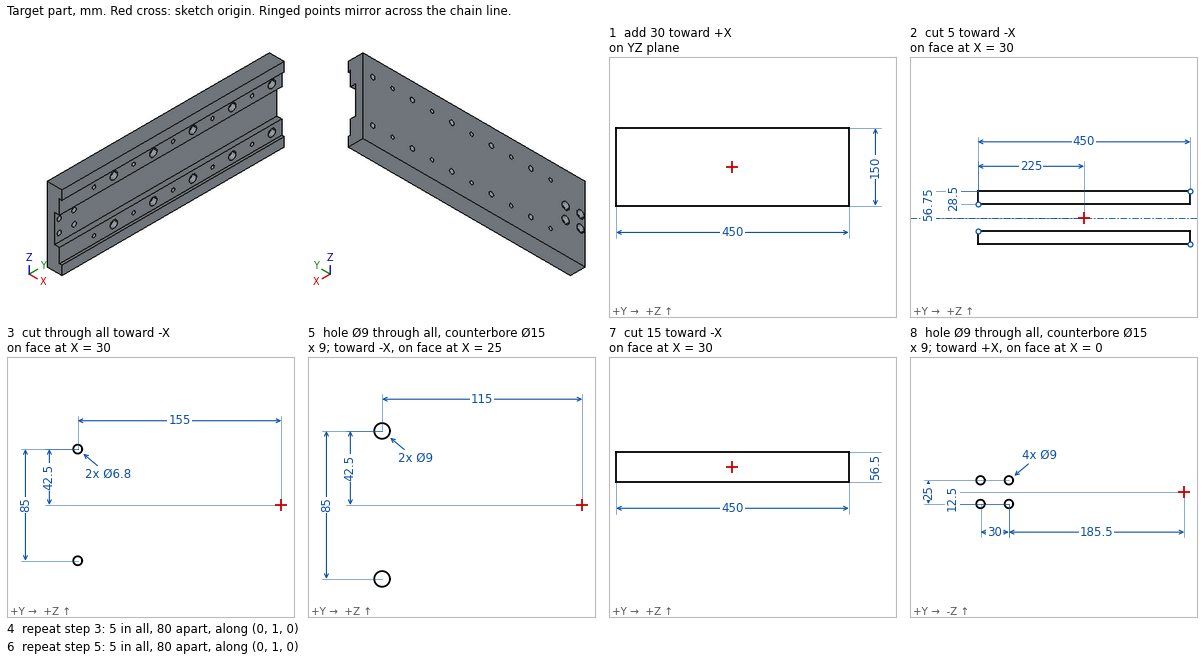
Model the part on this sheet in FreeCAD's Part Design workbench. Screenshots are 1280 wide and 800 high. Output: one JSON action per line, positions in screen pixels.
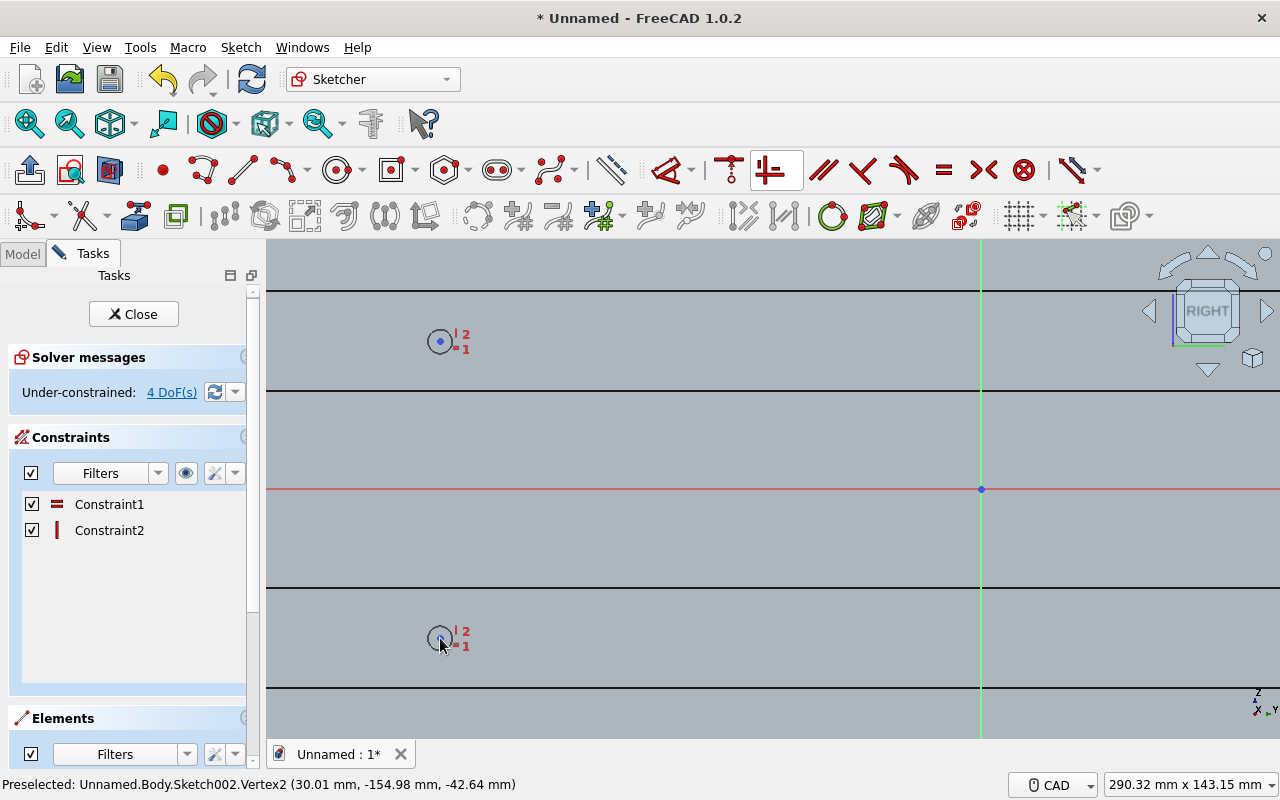
{"action": "left_click", "coordinate": [666, 170]}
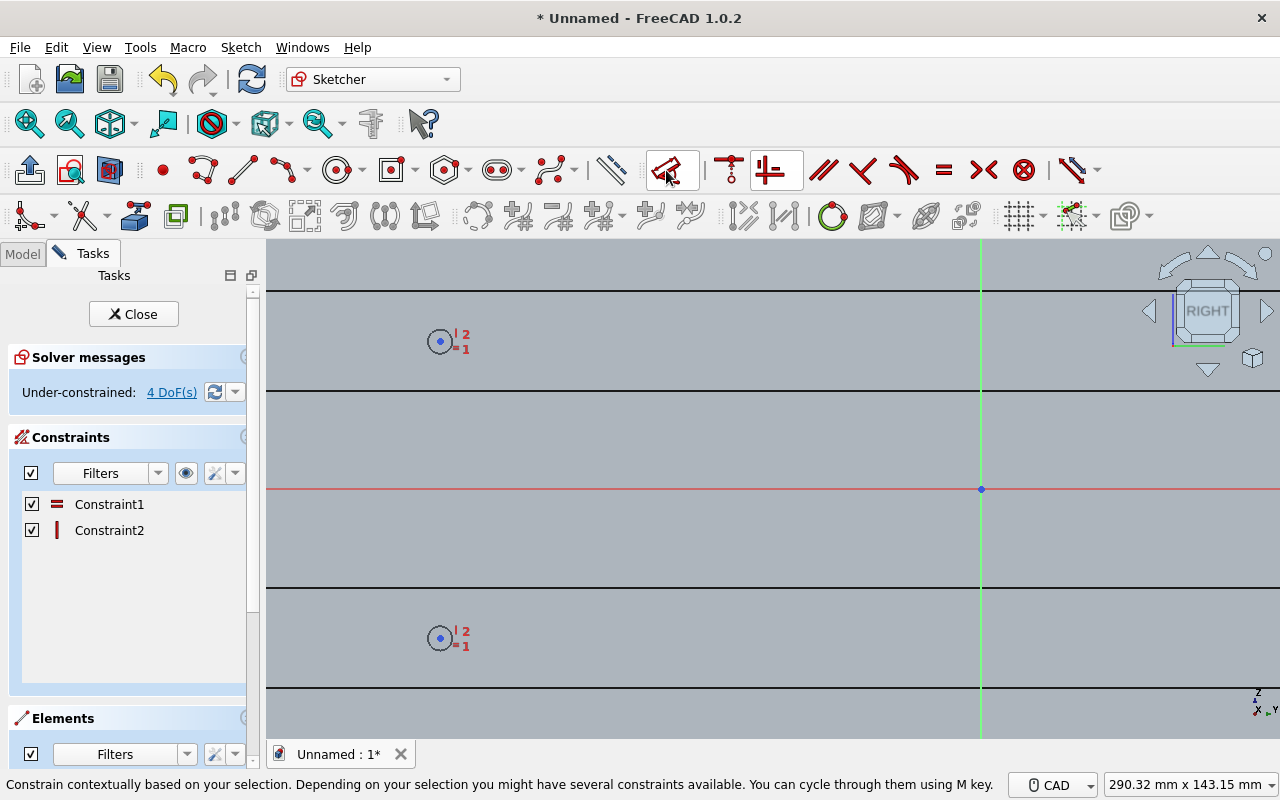
{"action": "scroll", "coordinate": [449, 333], "scroll_direction": "up", "scroll_amount": 3}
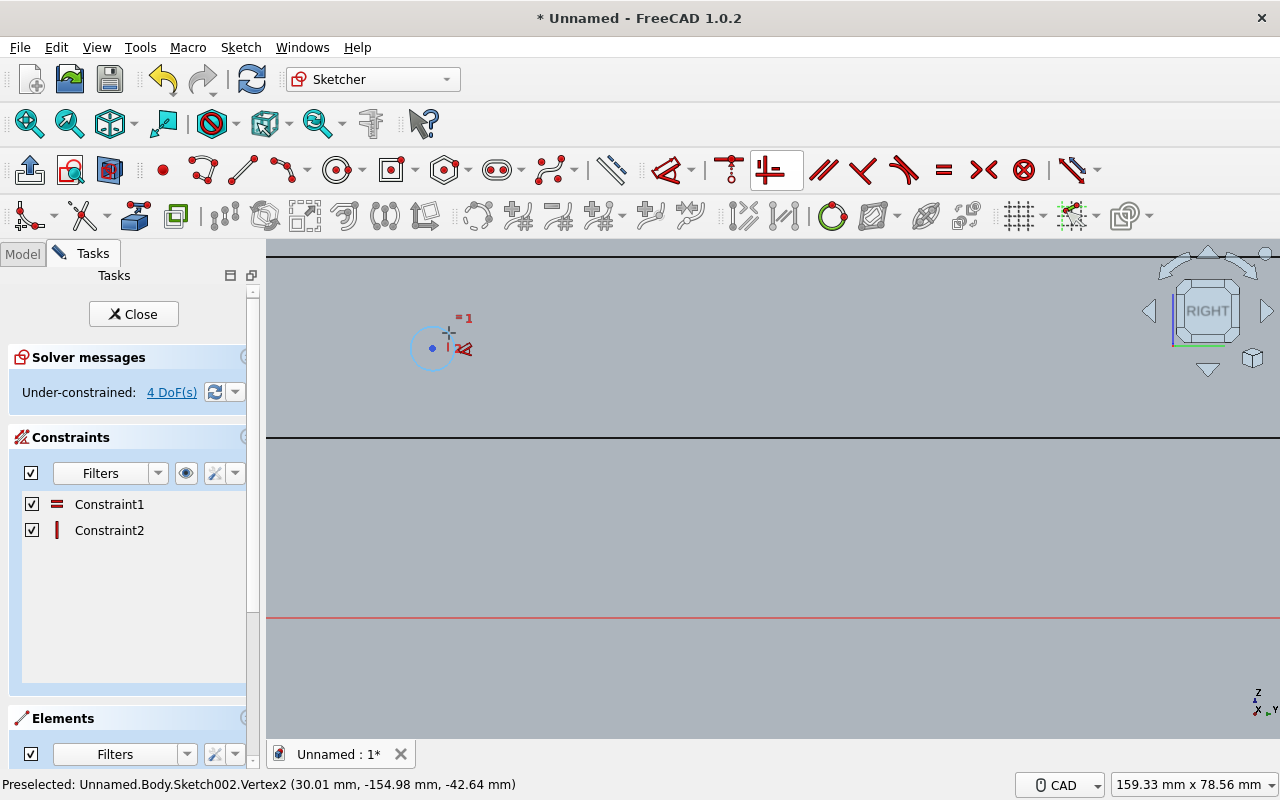
{"action": "left_click", "coordinate": [448, 333]}
{"action": "left_click", "coordinate": [470, 310]}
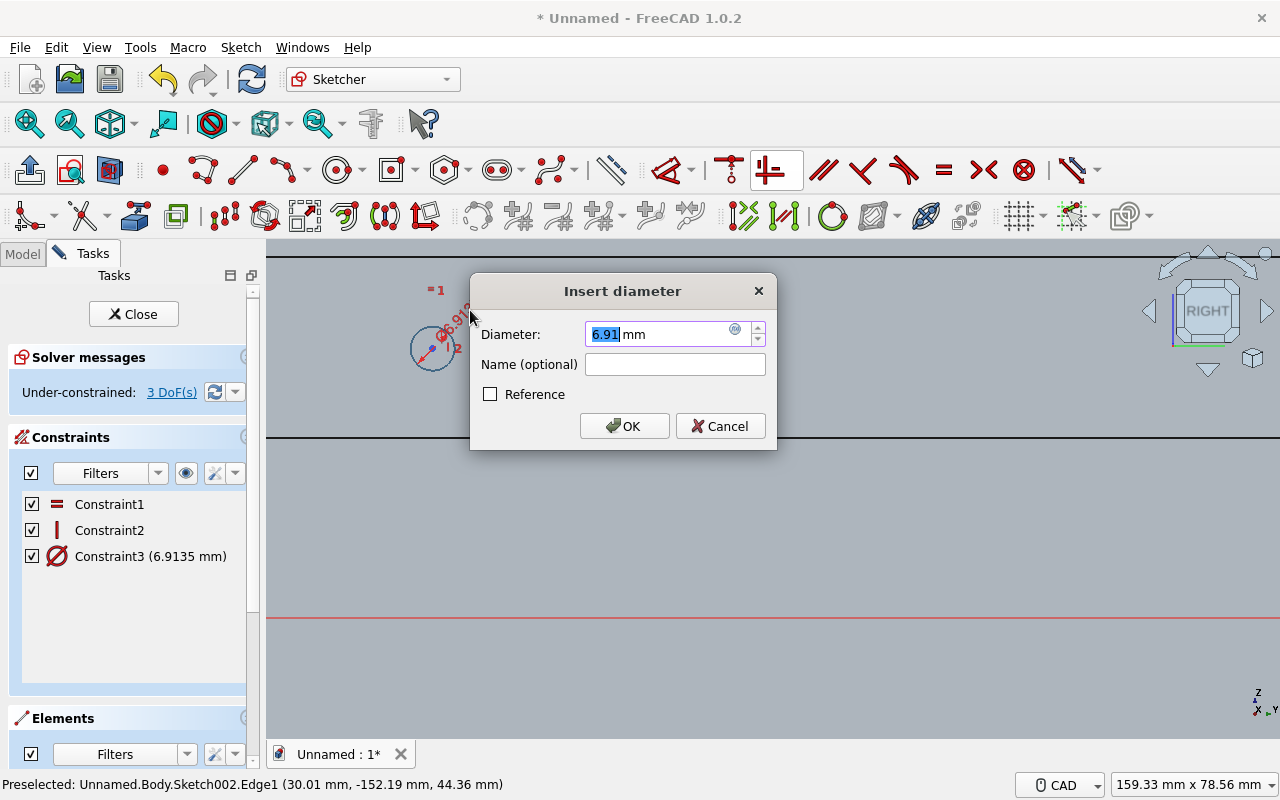
{"action": "type", "text": "6.8"}
{"action": "key", "text": "Return"}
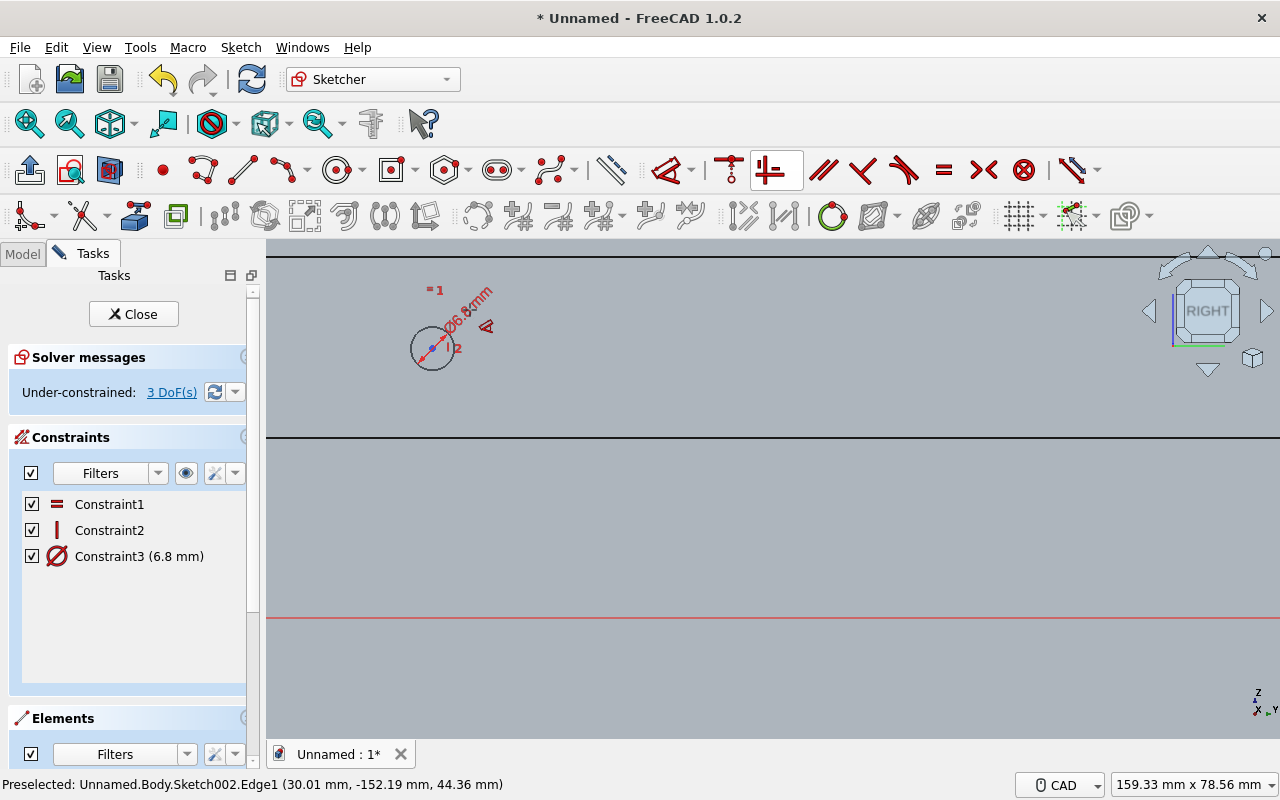
{"action": "left_click", "coordinate": [433, 349]}
{"action": "left_click", "coordinate": [774, 315]}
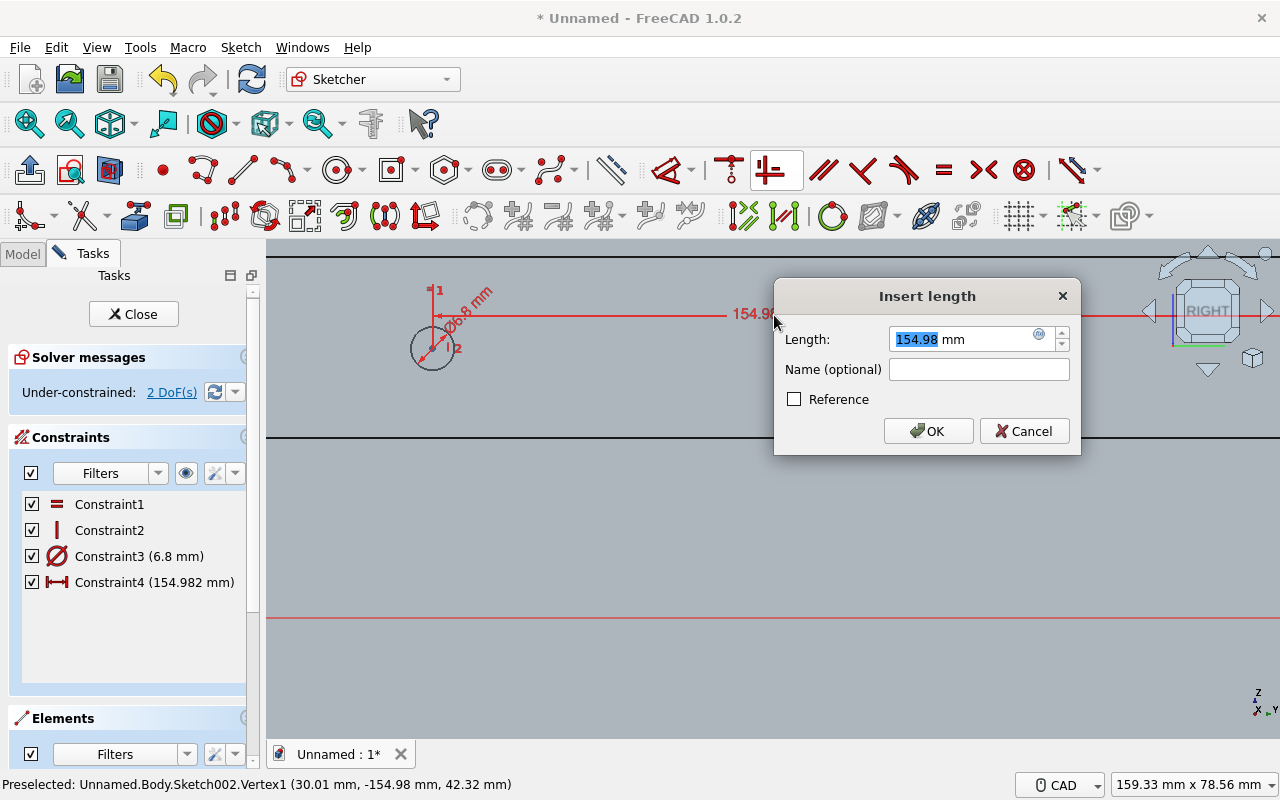
{"action": "type", "text": "155"}
{"action": "key", "text": "Return"}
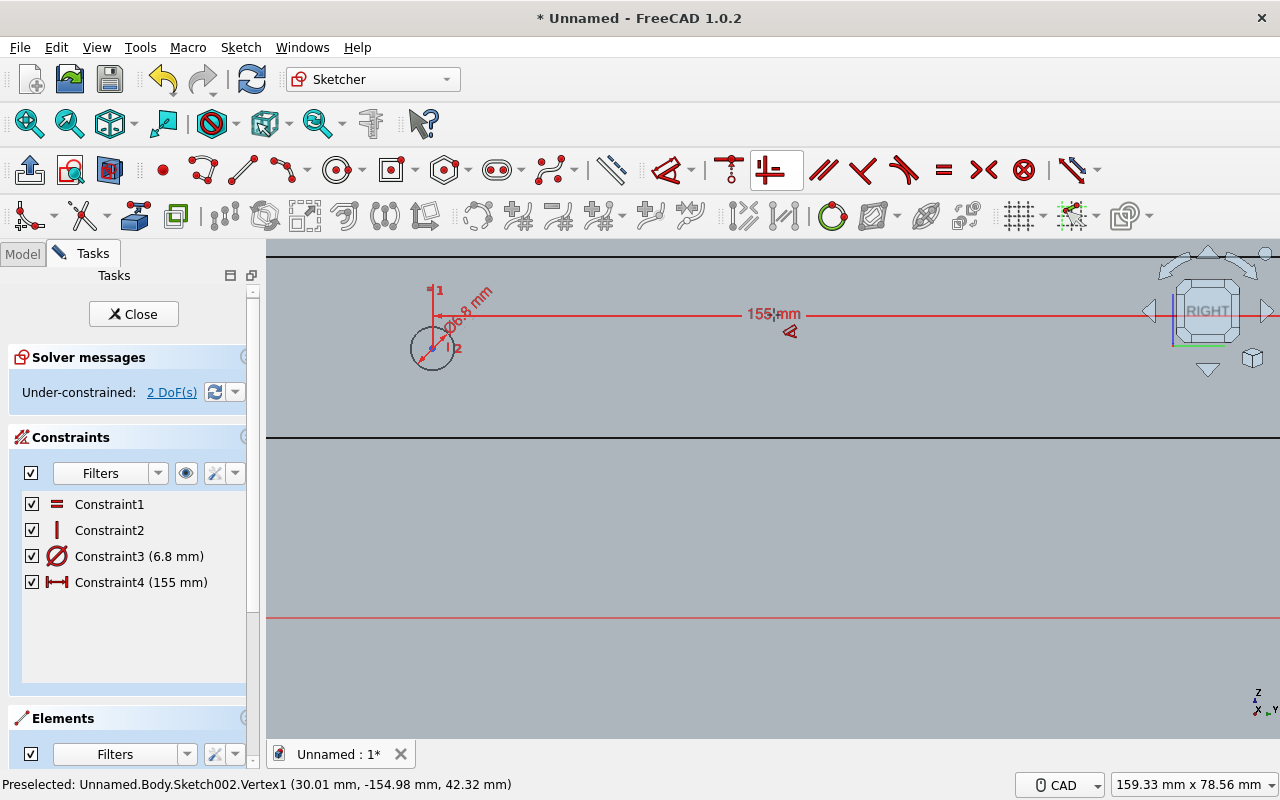
{"action": "left_click", "coordinate": [433, 349]}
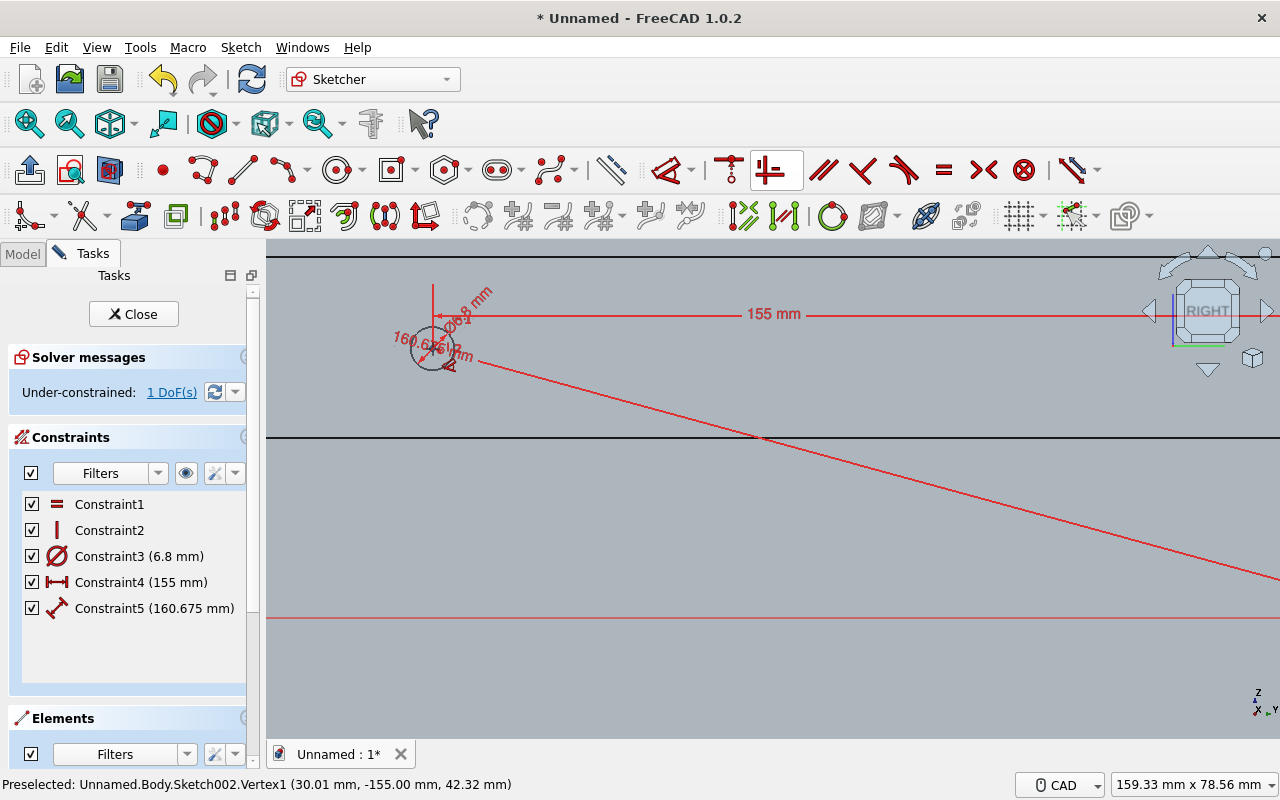
{"action": "scroll", "coordinate": [449, 332], "scroll_direction": "down", "scroll_amount": 3}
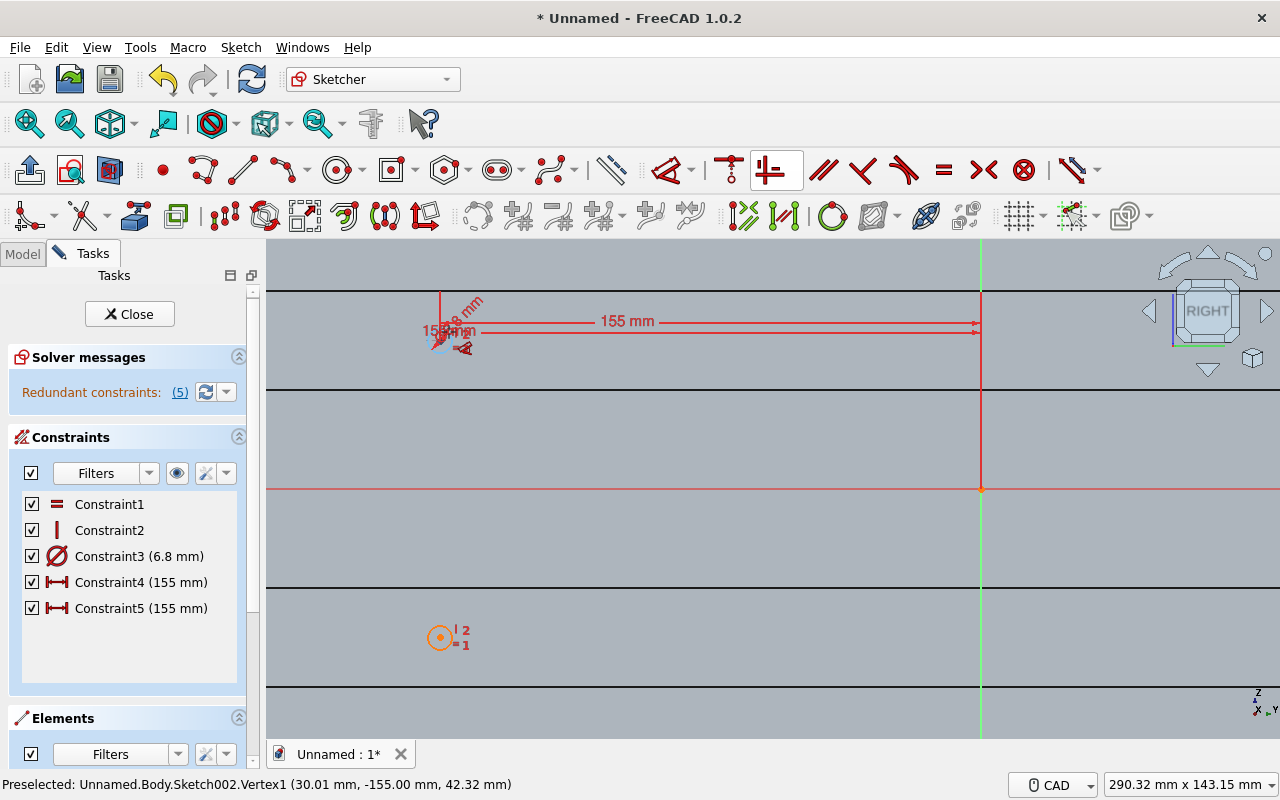
{"action": "left_click", "coordinate": [440, 638]}
{"action": "left_click", "coordinate": [406, 421]}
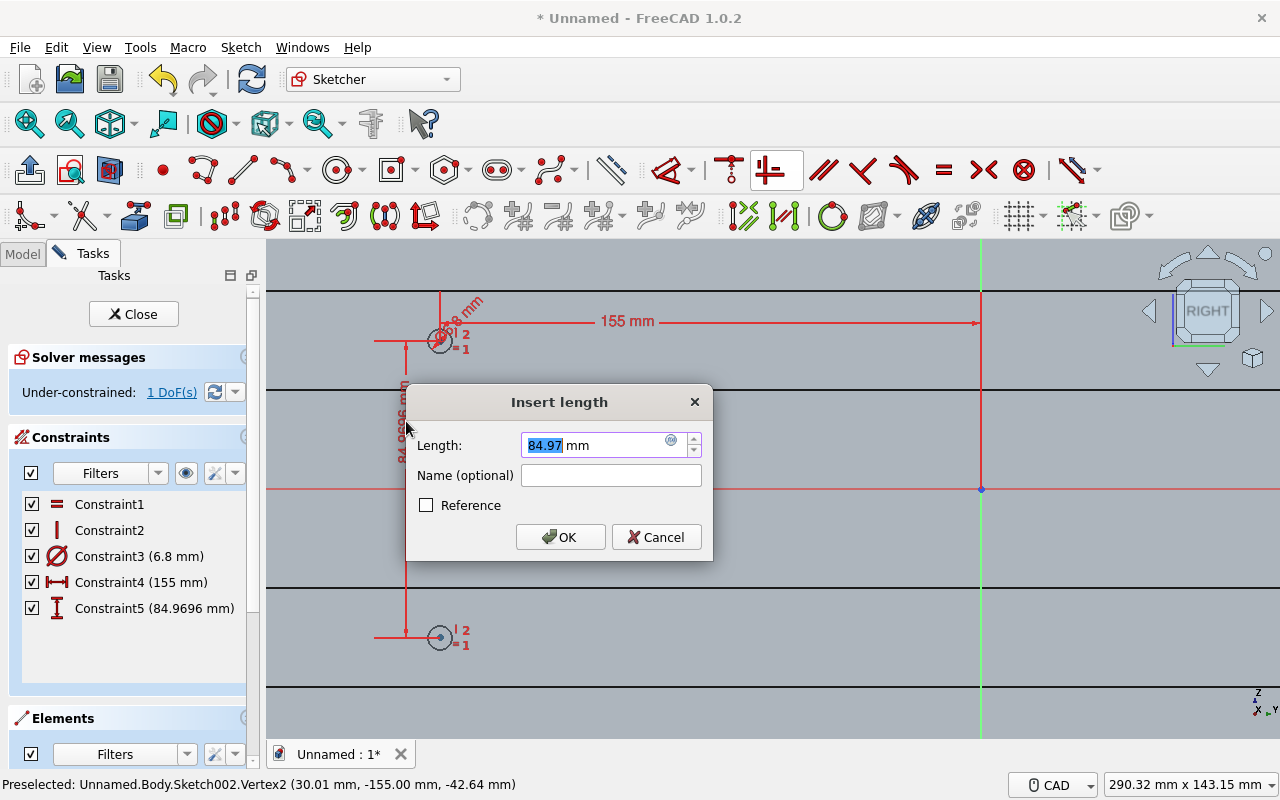
{"action": "type", "text": "85"}
{"action": "key", "text": "Return"}